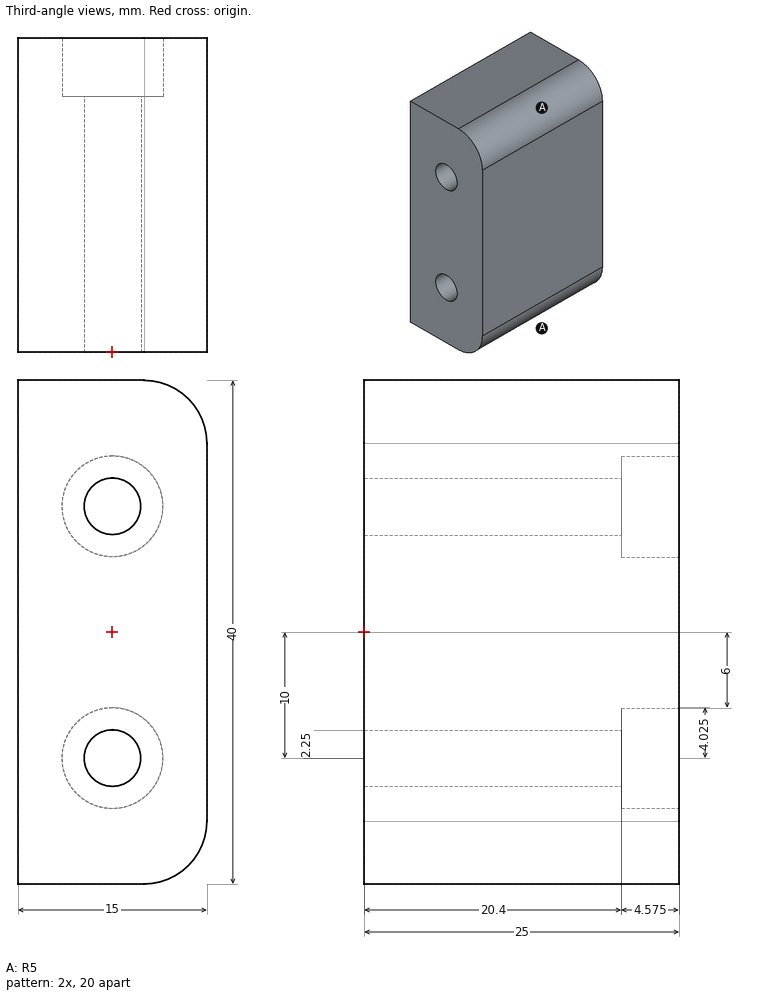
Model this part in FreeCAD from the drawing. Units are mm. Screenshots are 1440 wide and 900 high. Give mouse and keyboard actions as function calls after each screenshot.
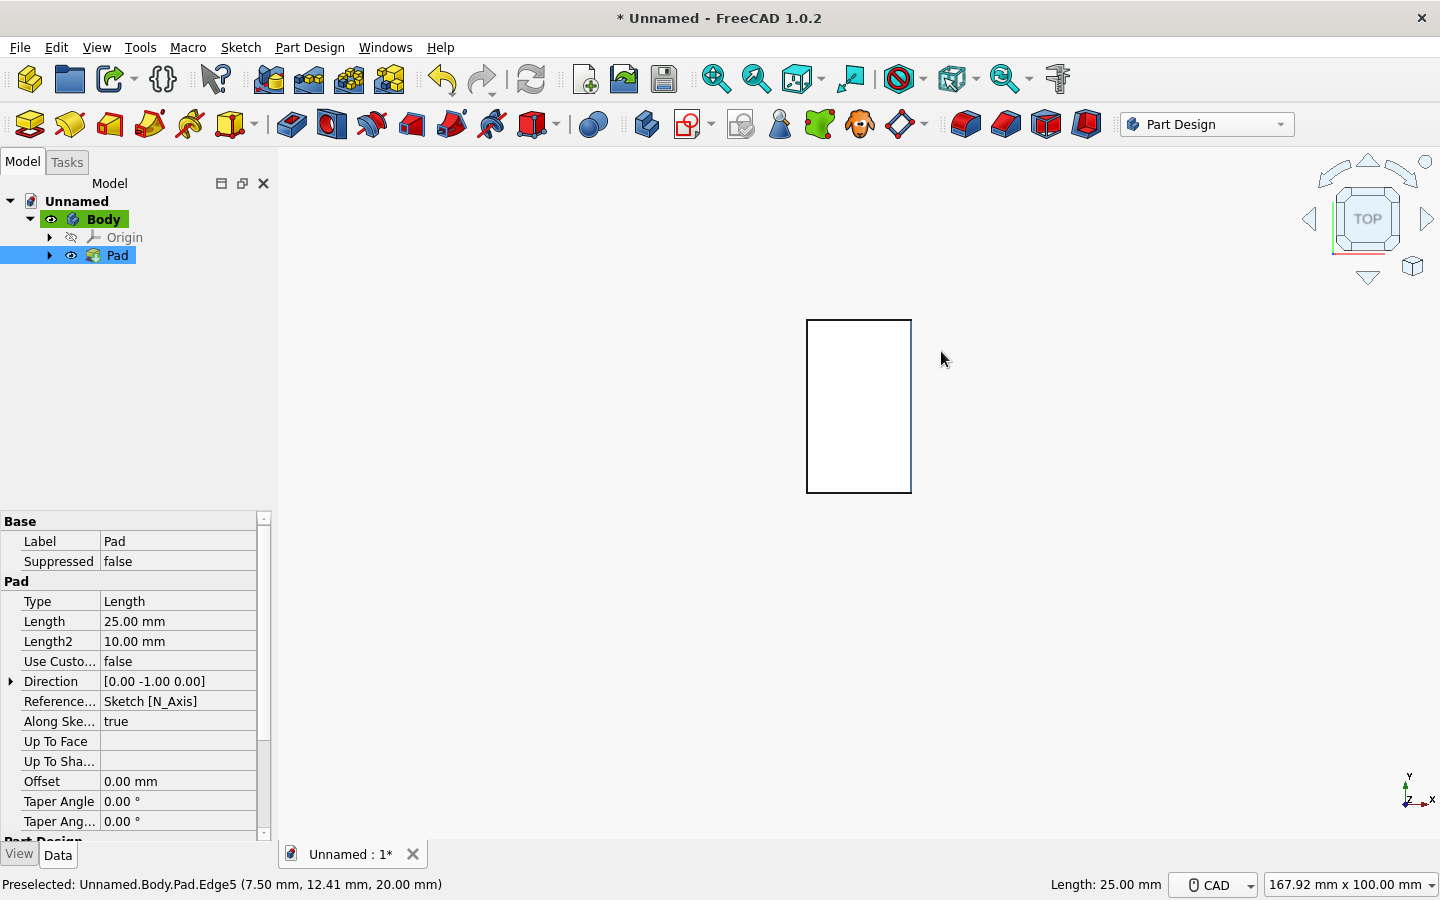
click(718, 80)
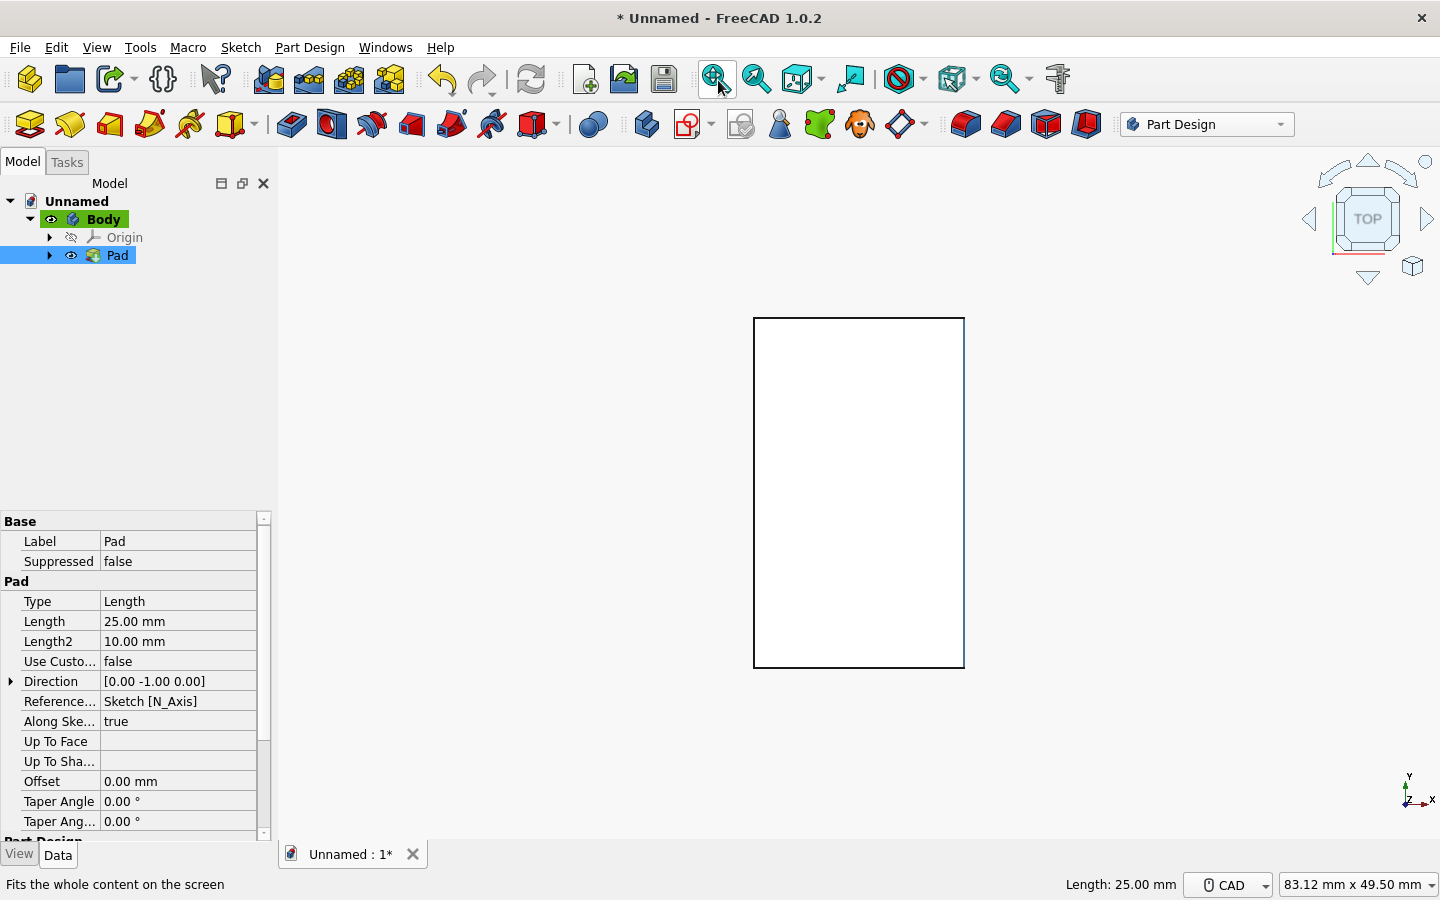
key(1)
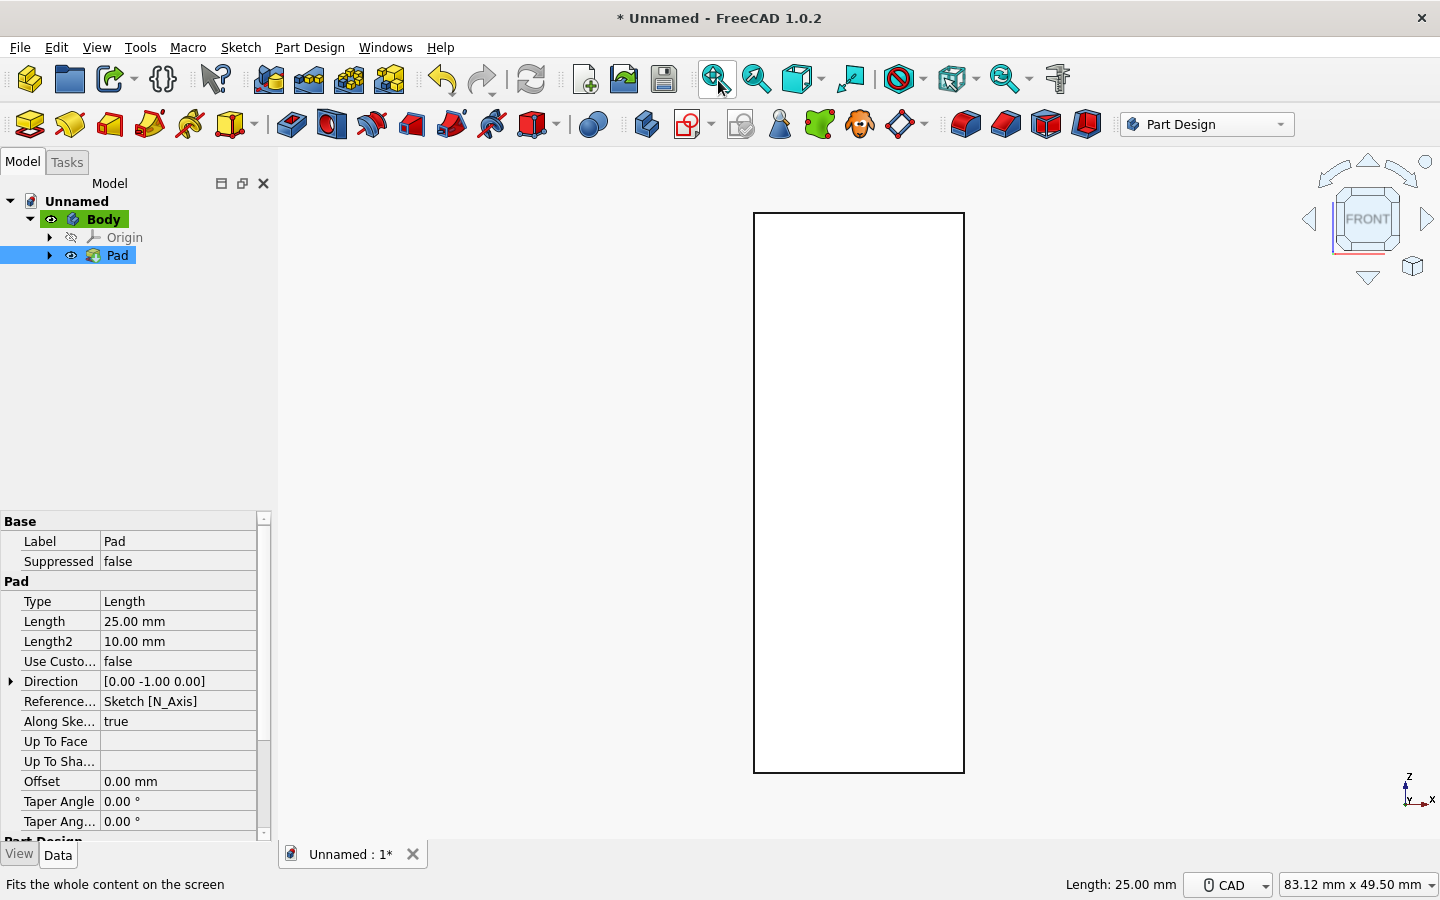
key(3)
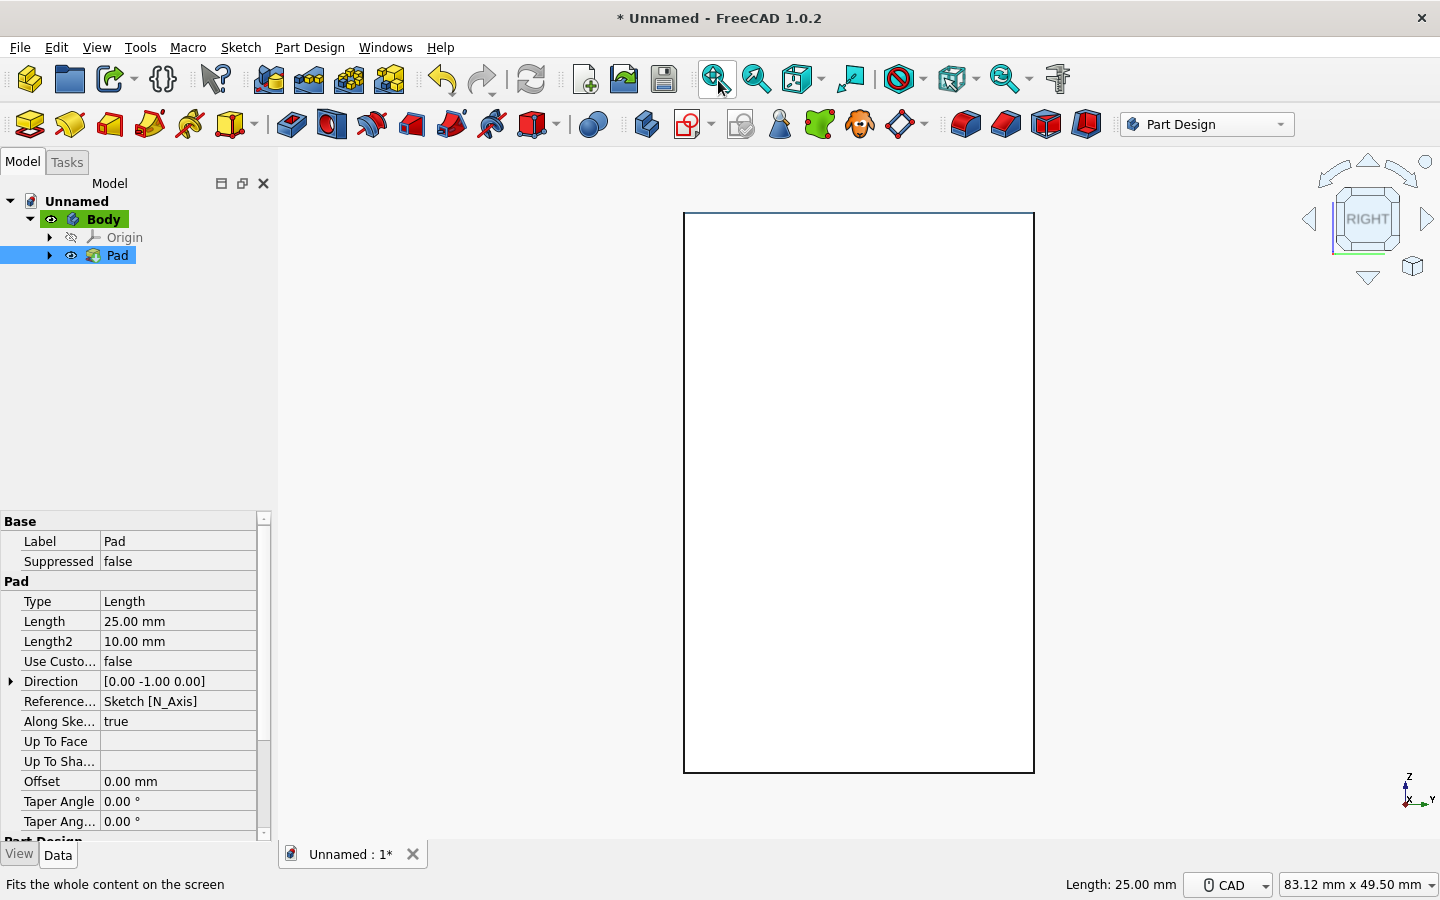
click(859, 772, ctrl)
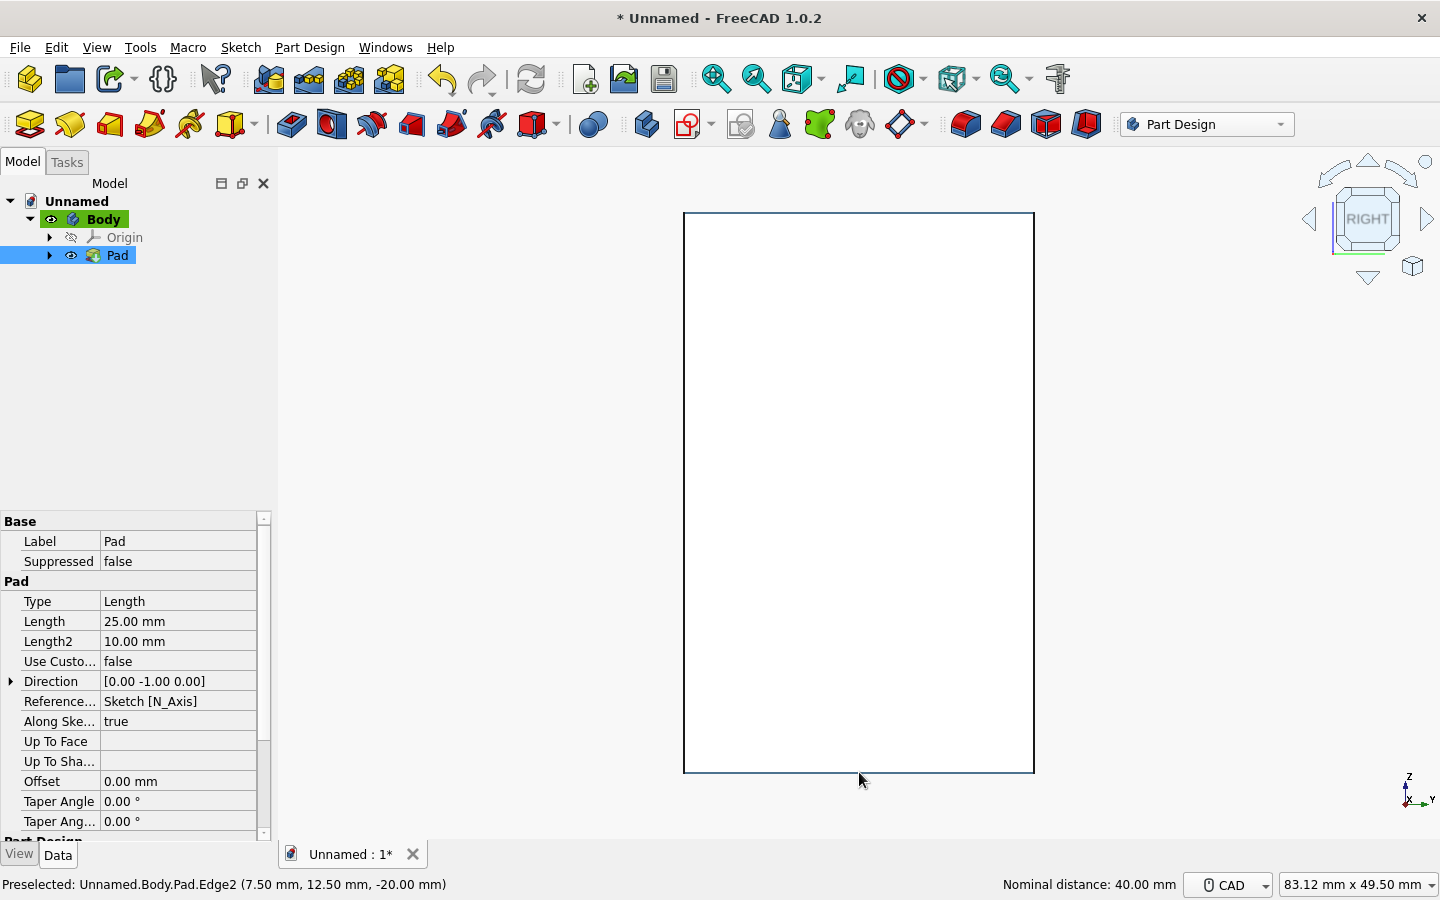
click(966, 124)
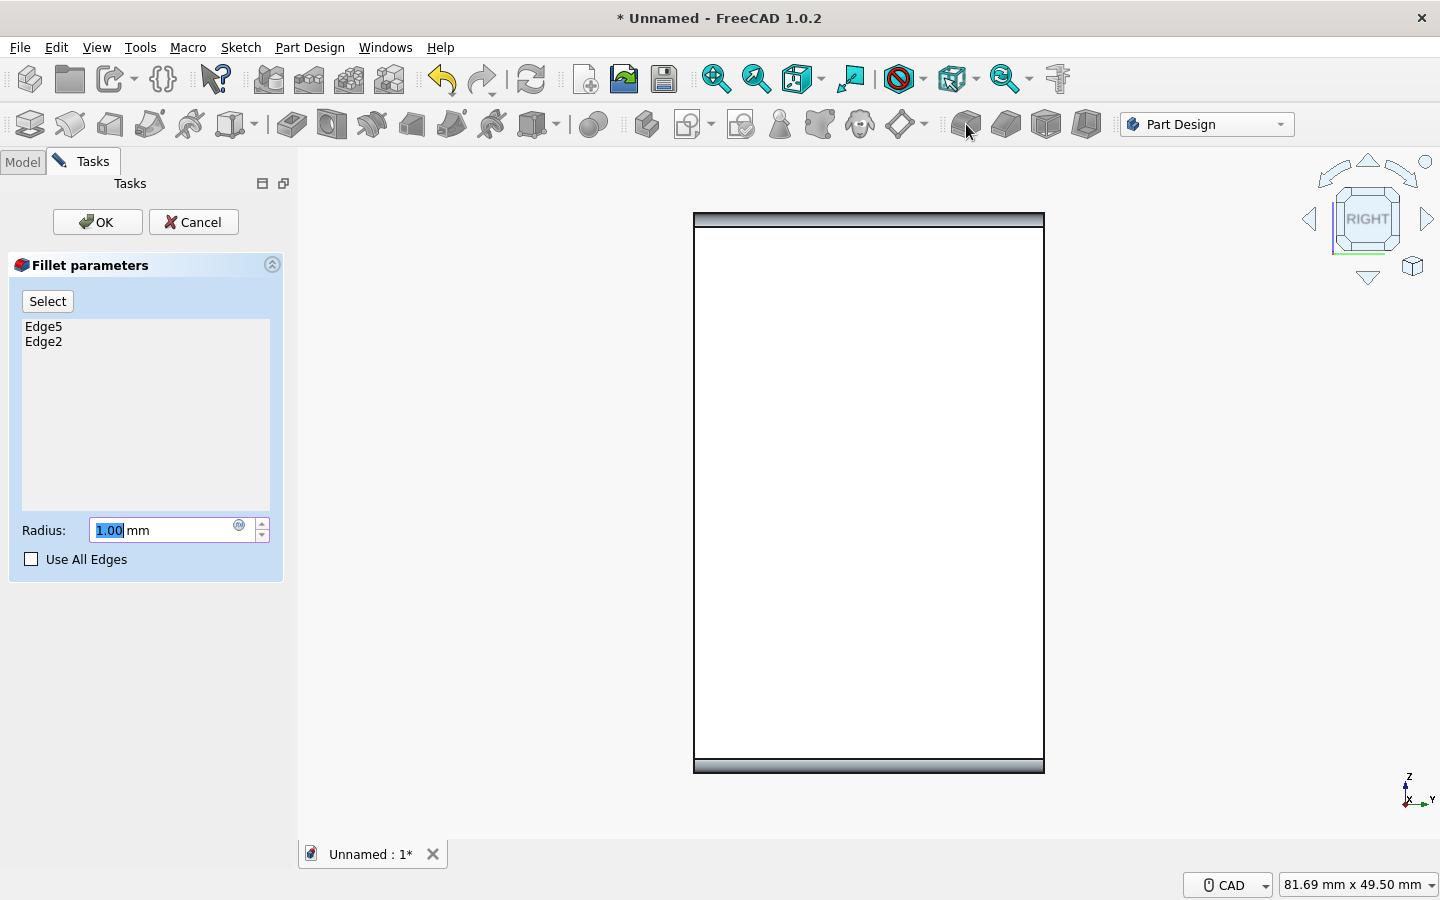
text(5)
key(Tab)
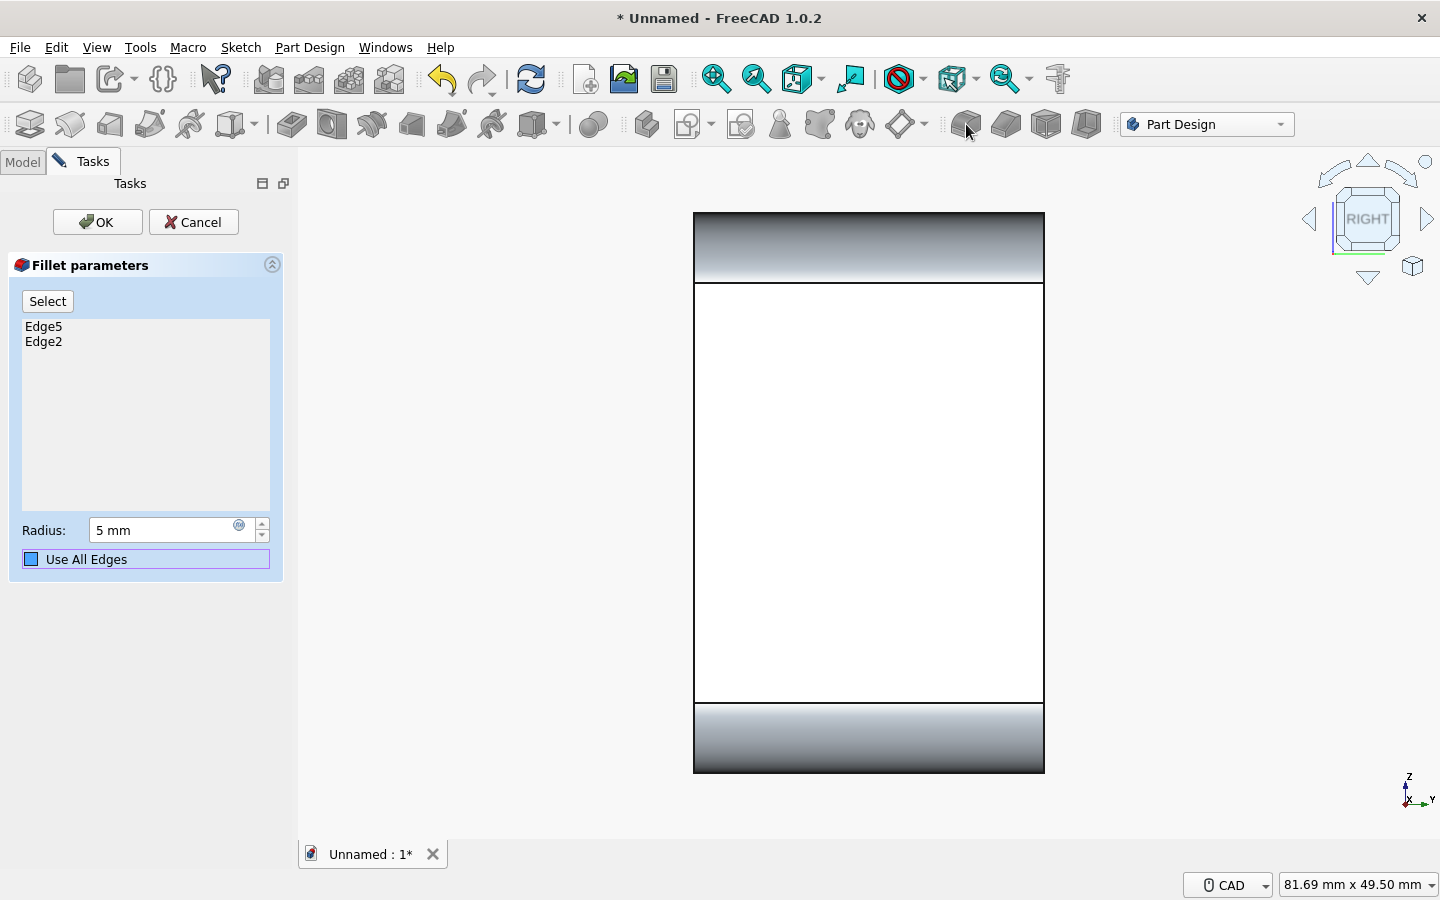
click(98, 222)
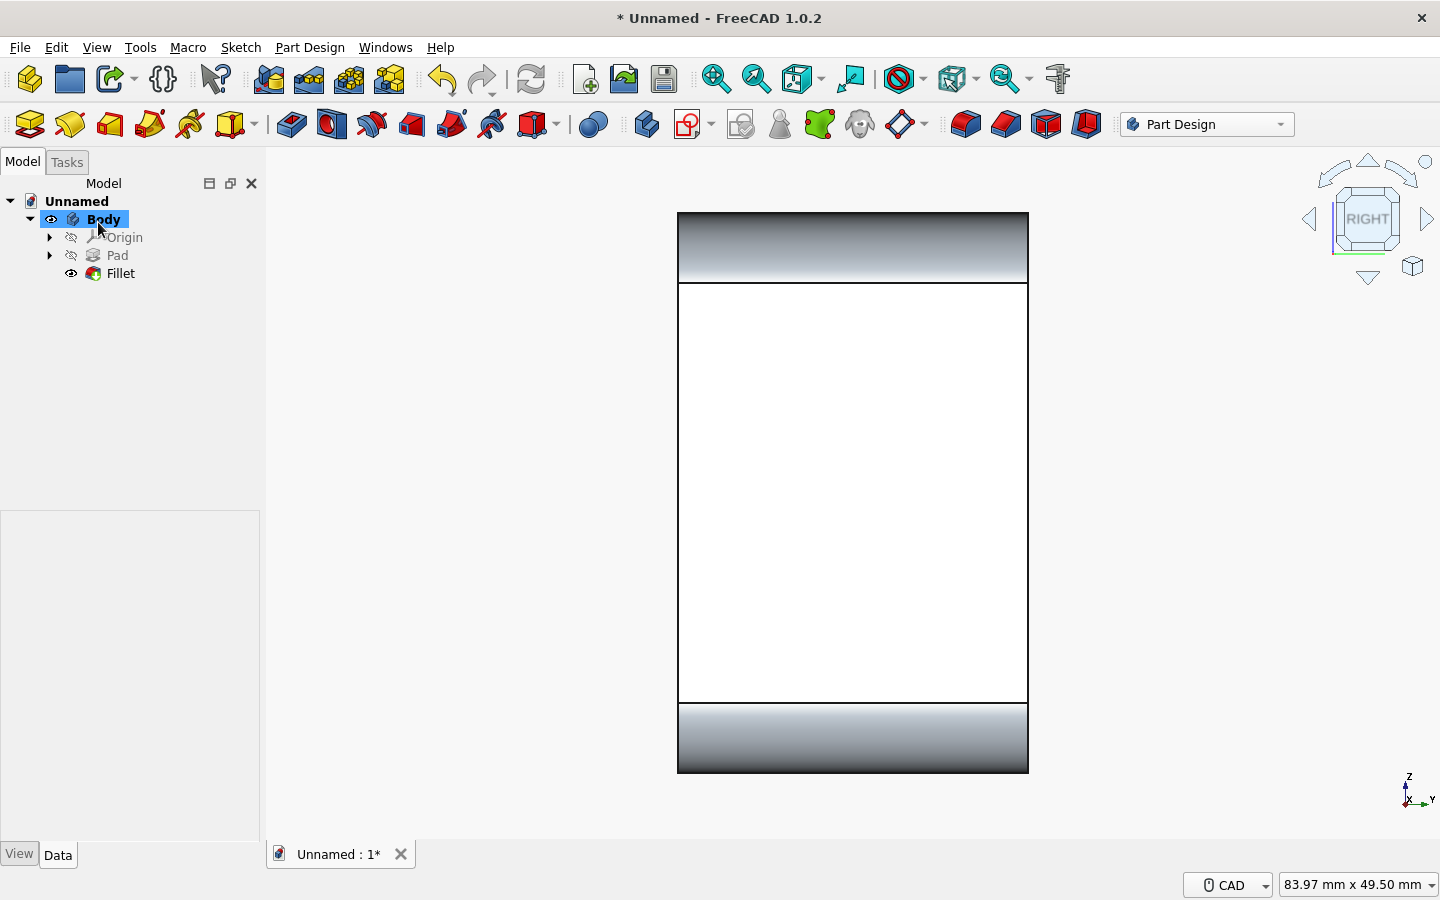
click(688, 124)